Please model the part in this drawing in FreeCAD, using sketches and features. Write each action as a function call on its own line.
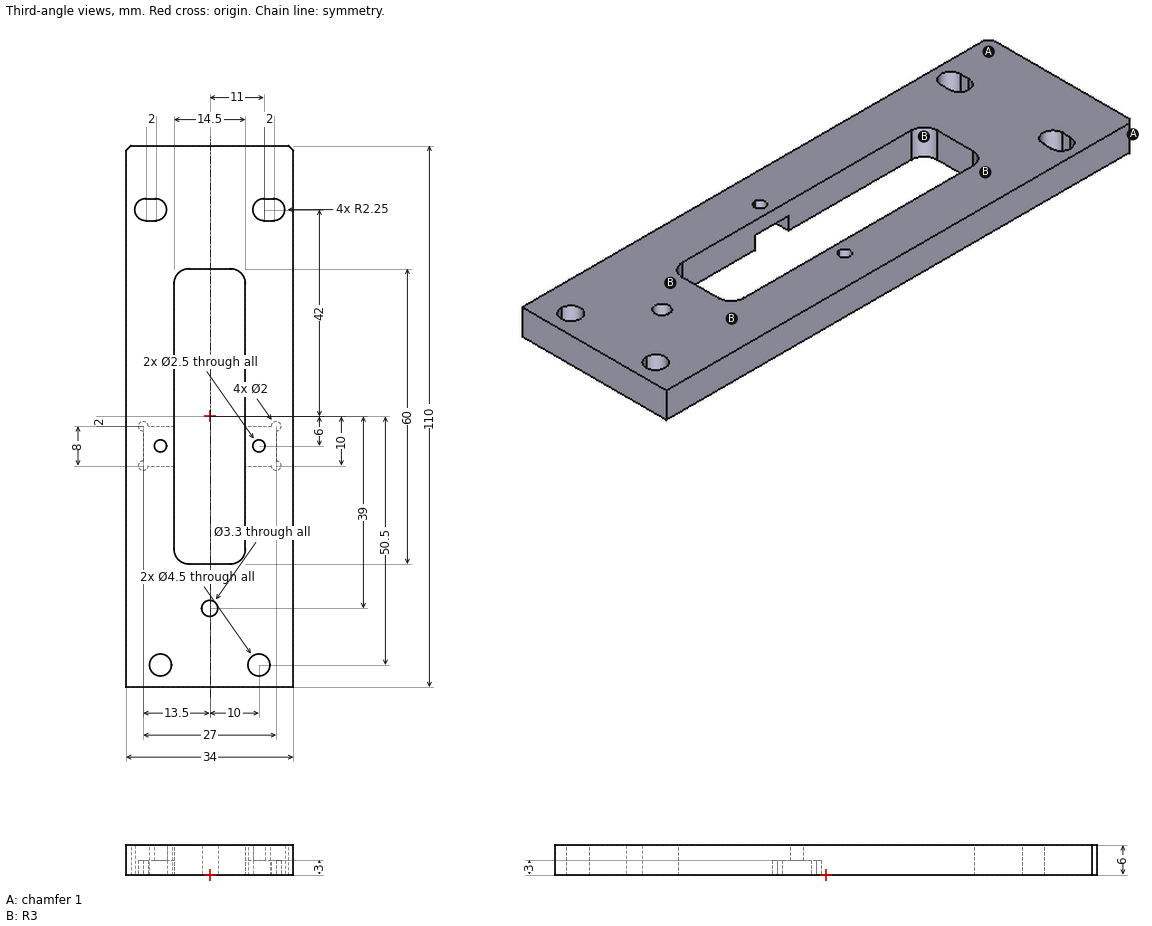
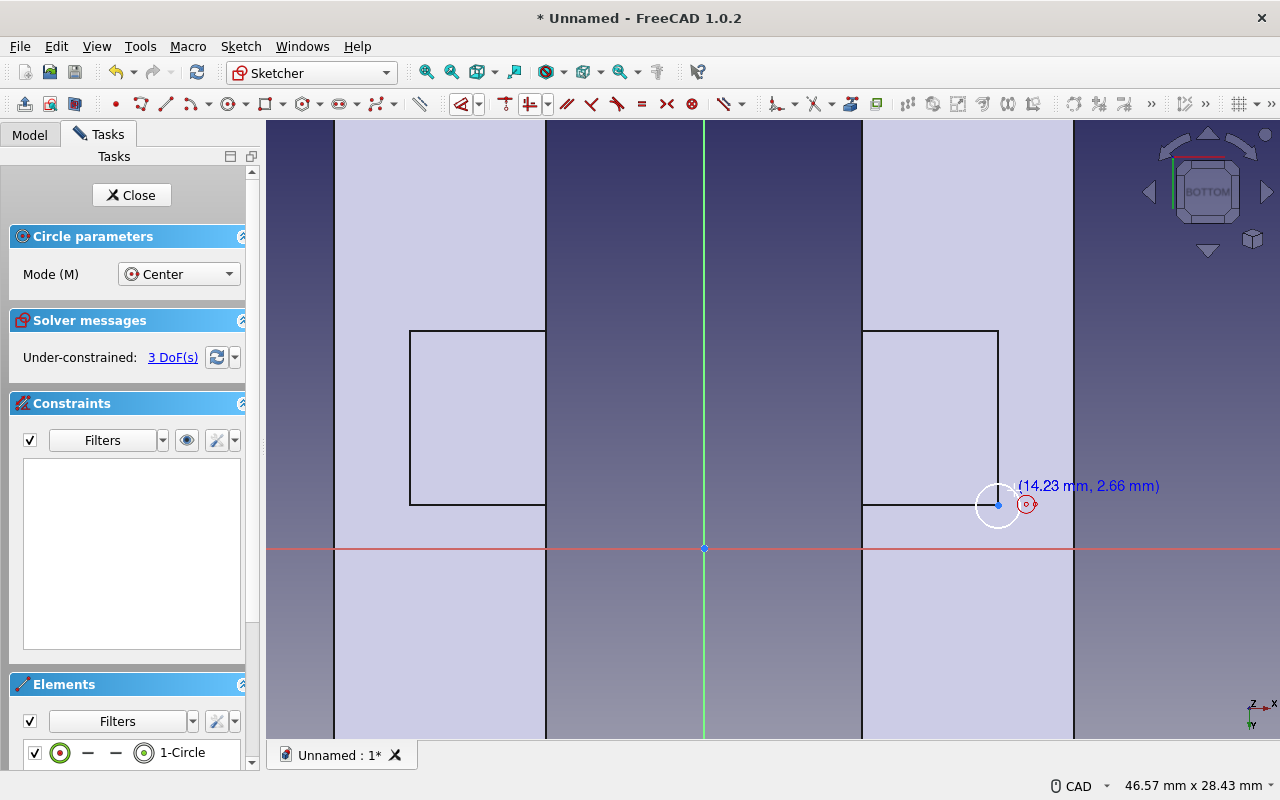
click(998, 331)
click(1014, 316)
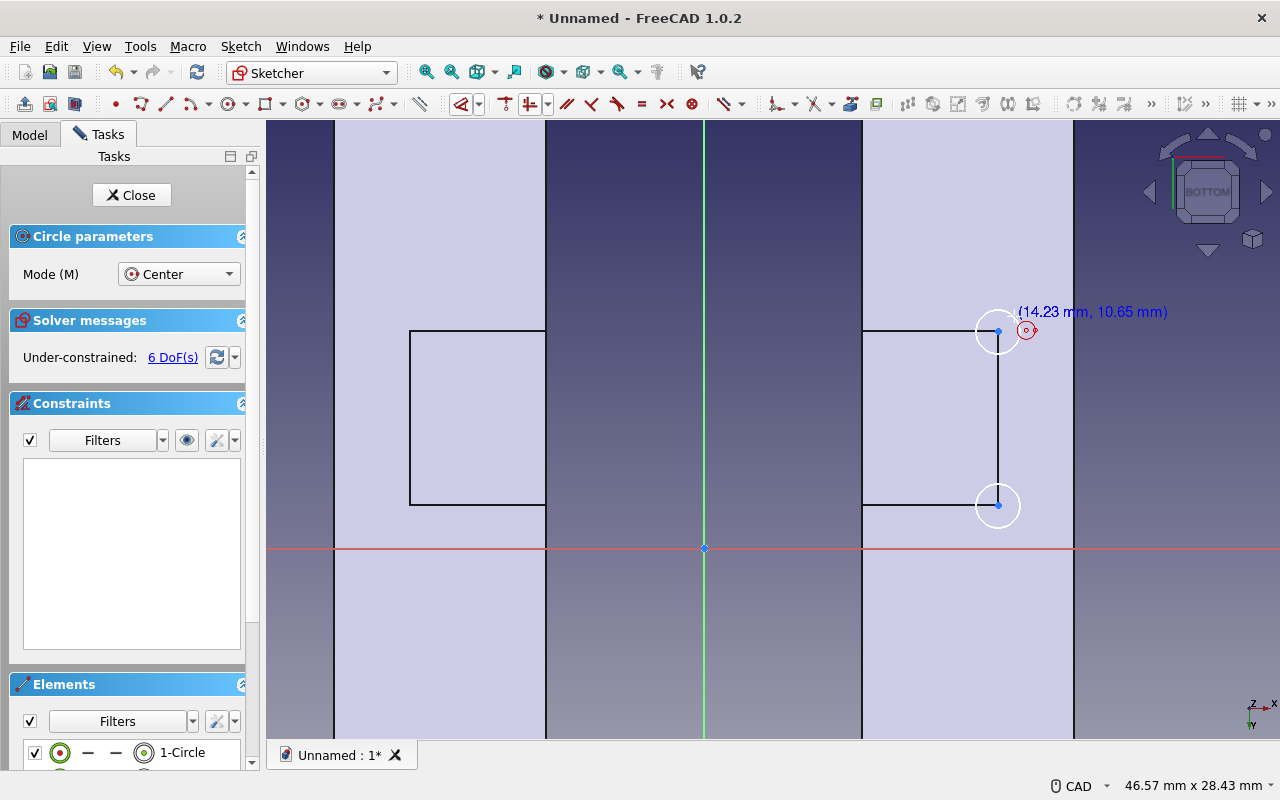
click(410, 331)
click(426, 316)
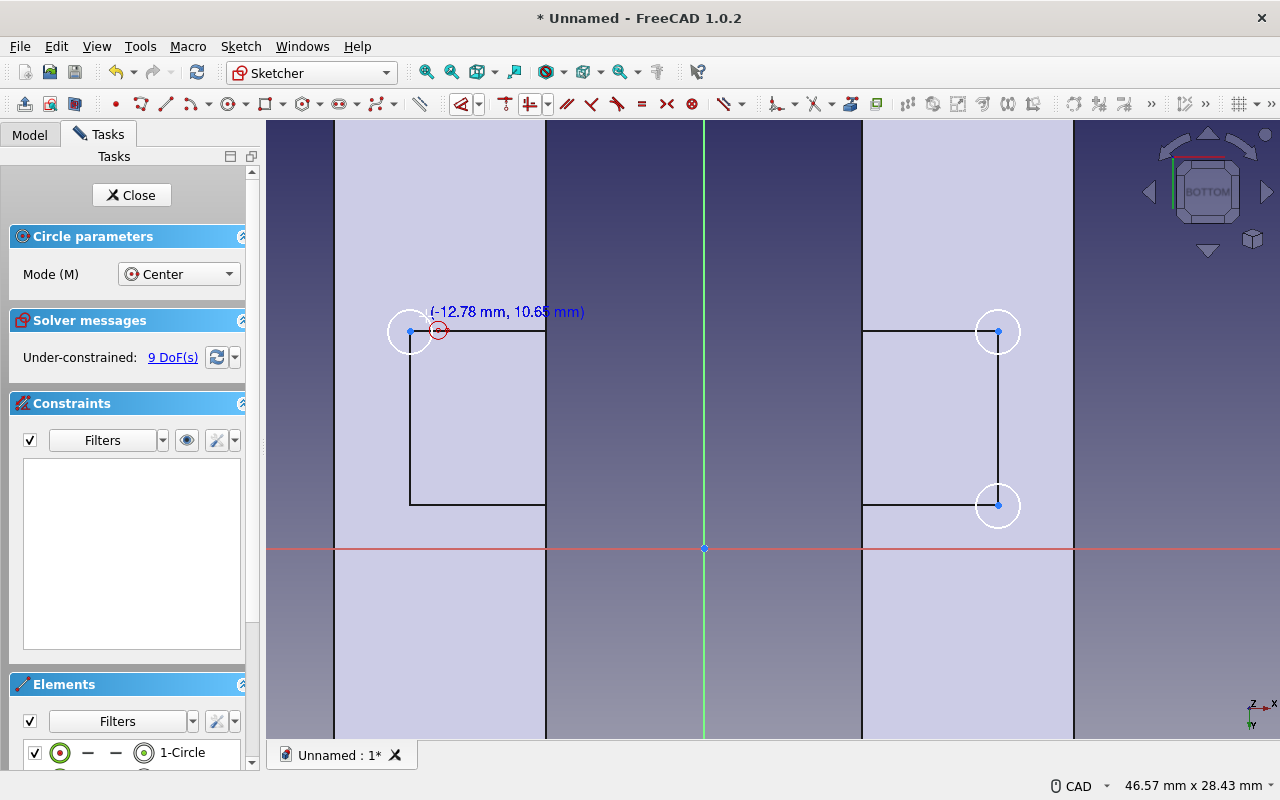
click(410, 505)
click(426, 490)
key(Escape)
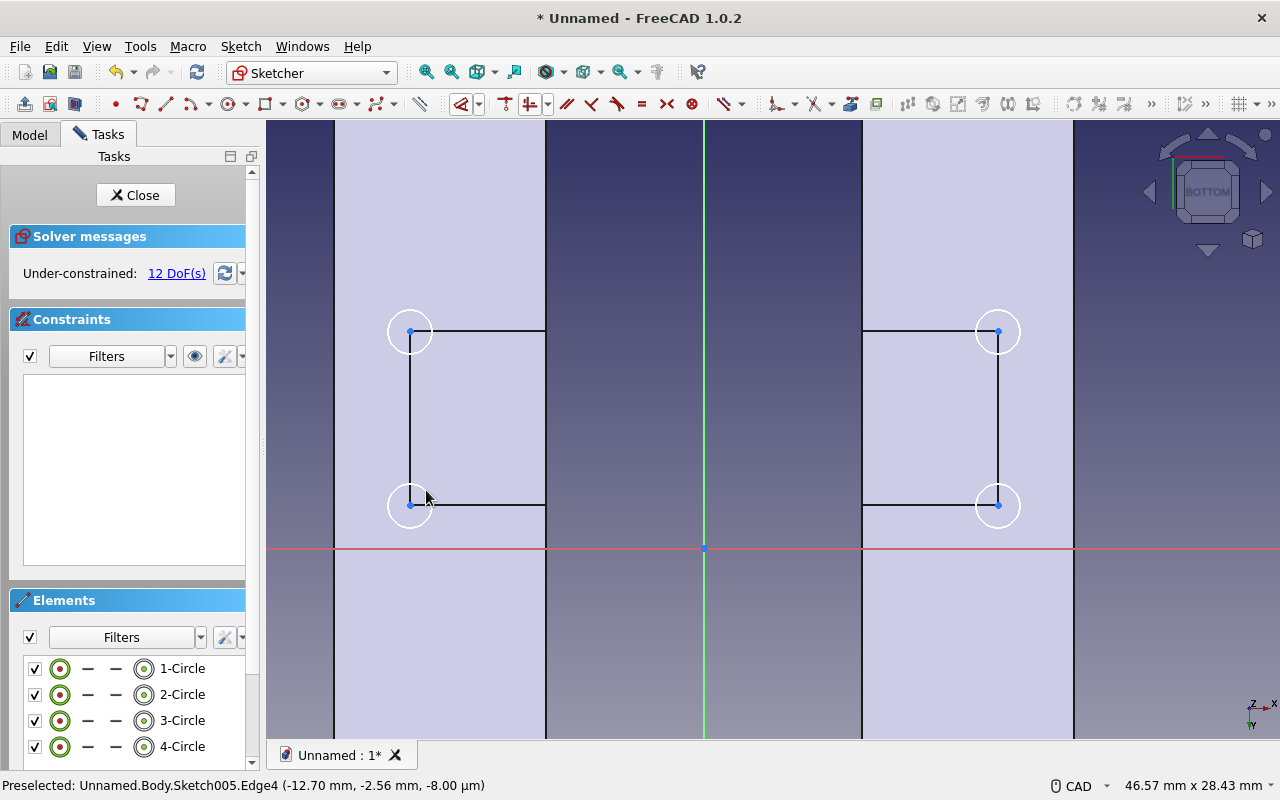
click(1013, 490)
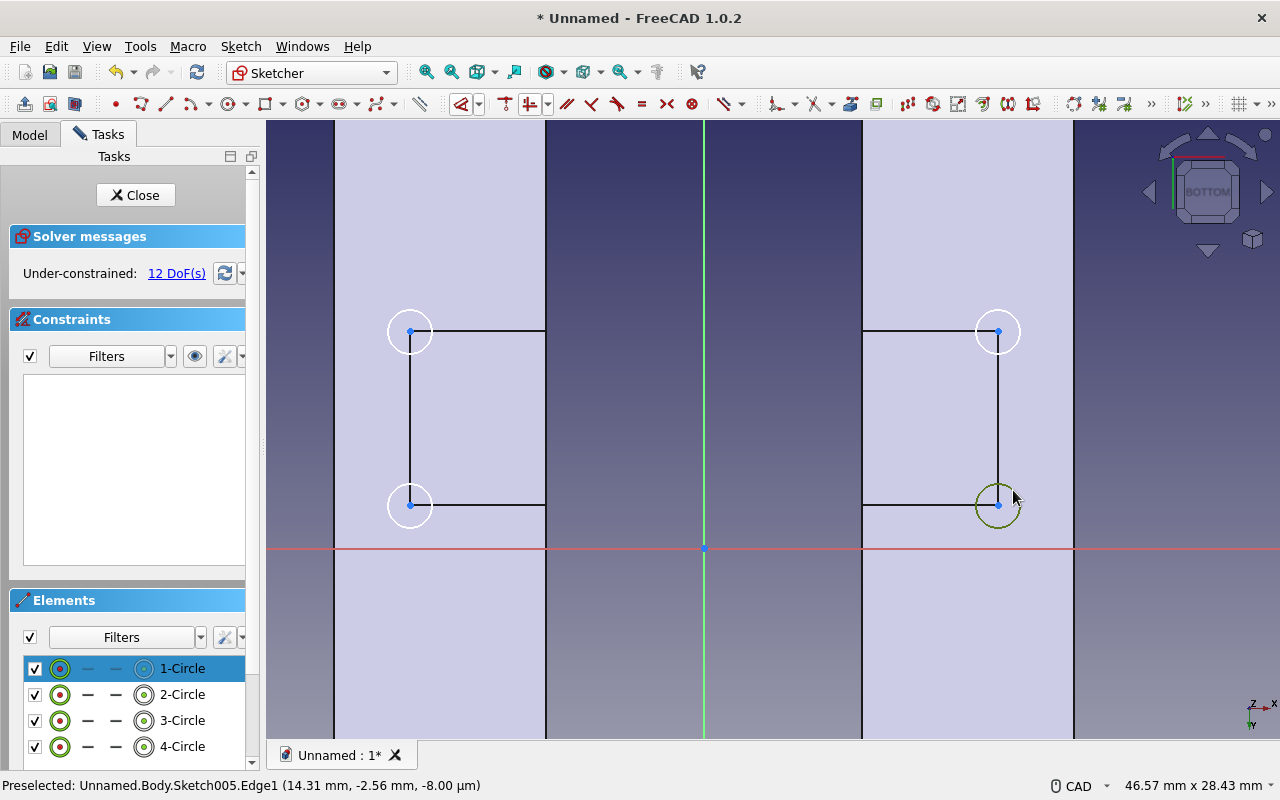
click(1013, 316)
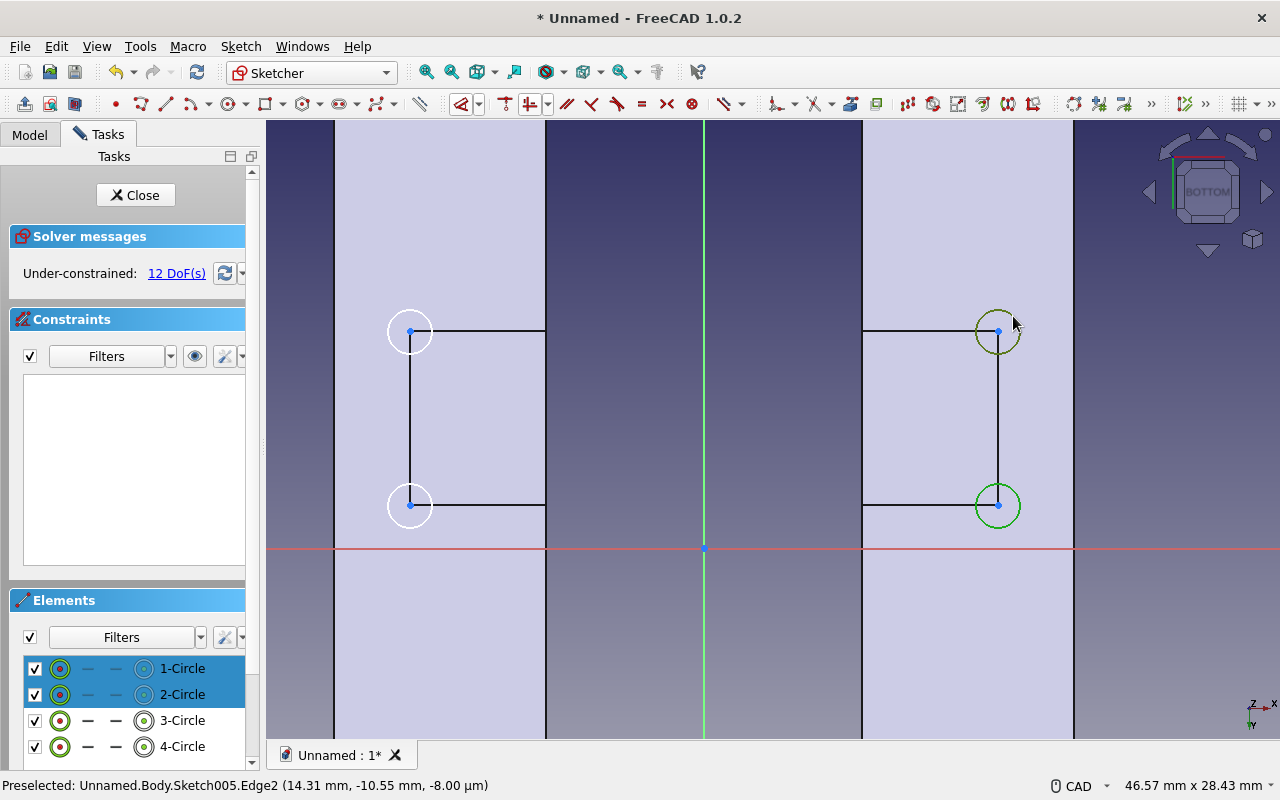
click(425, 316)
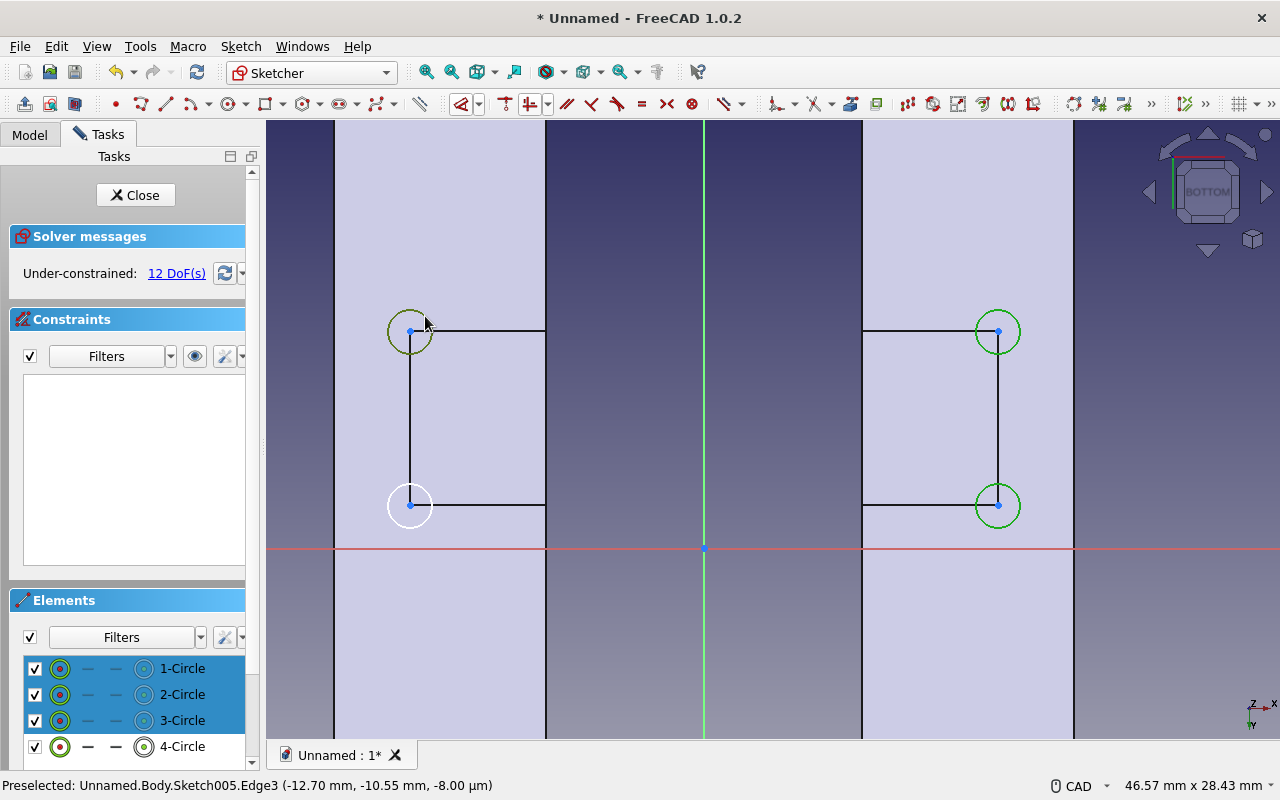
click(425, 490)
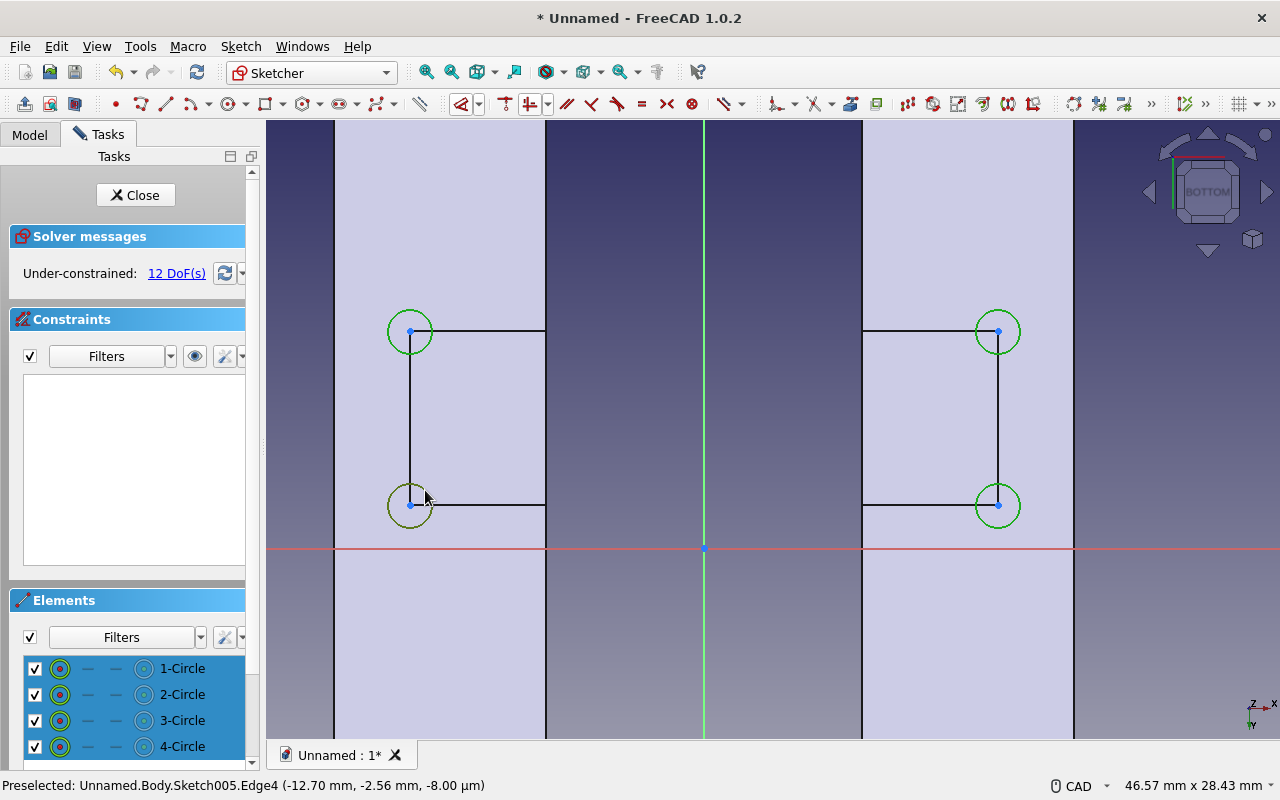
click(642, 104)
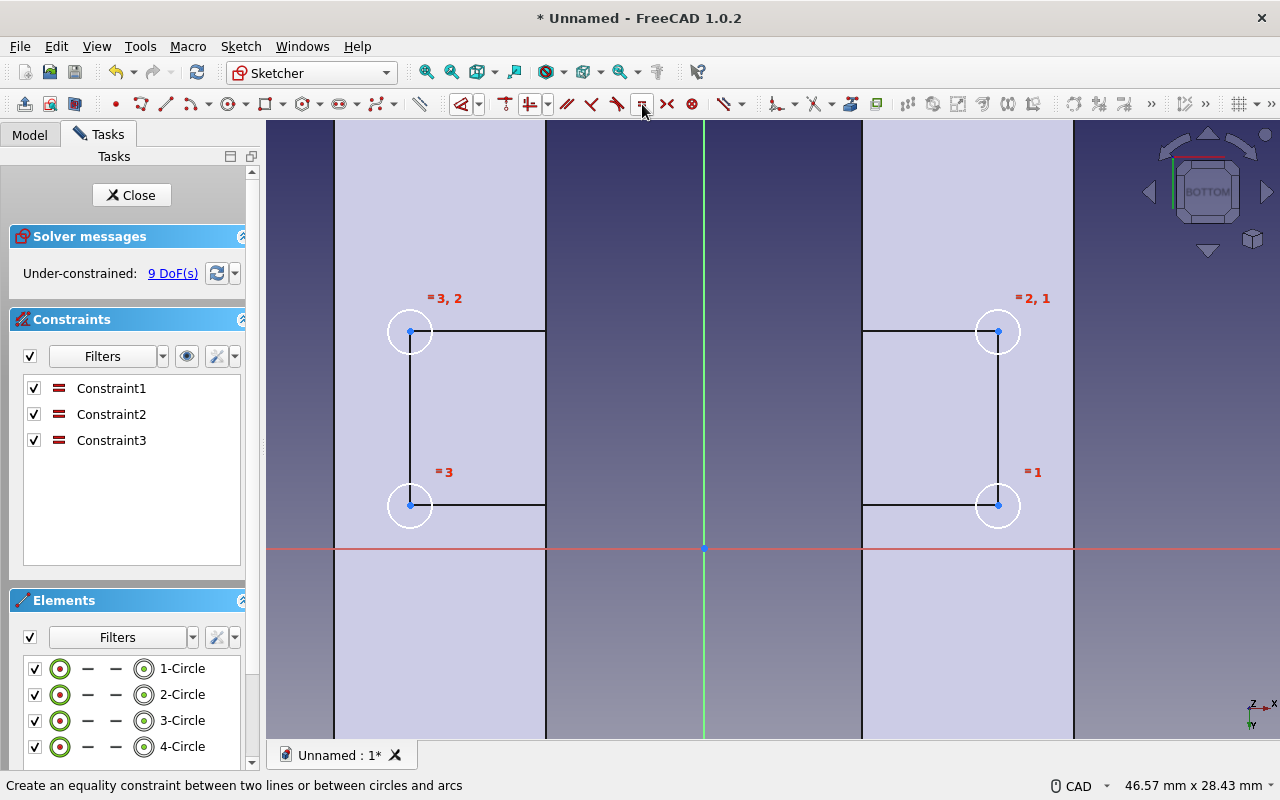
click(998, 332)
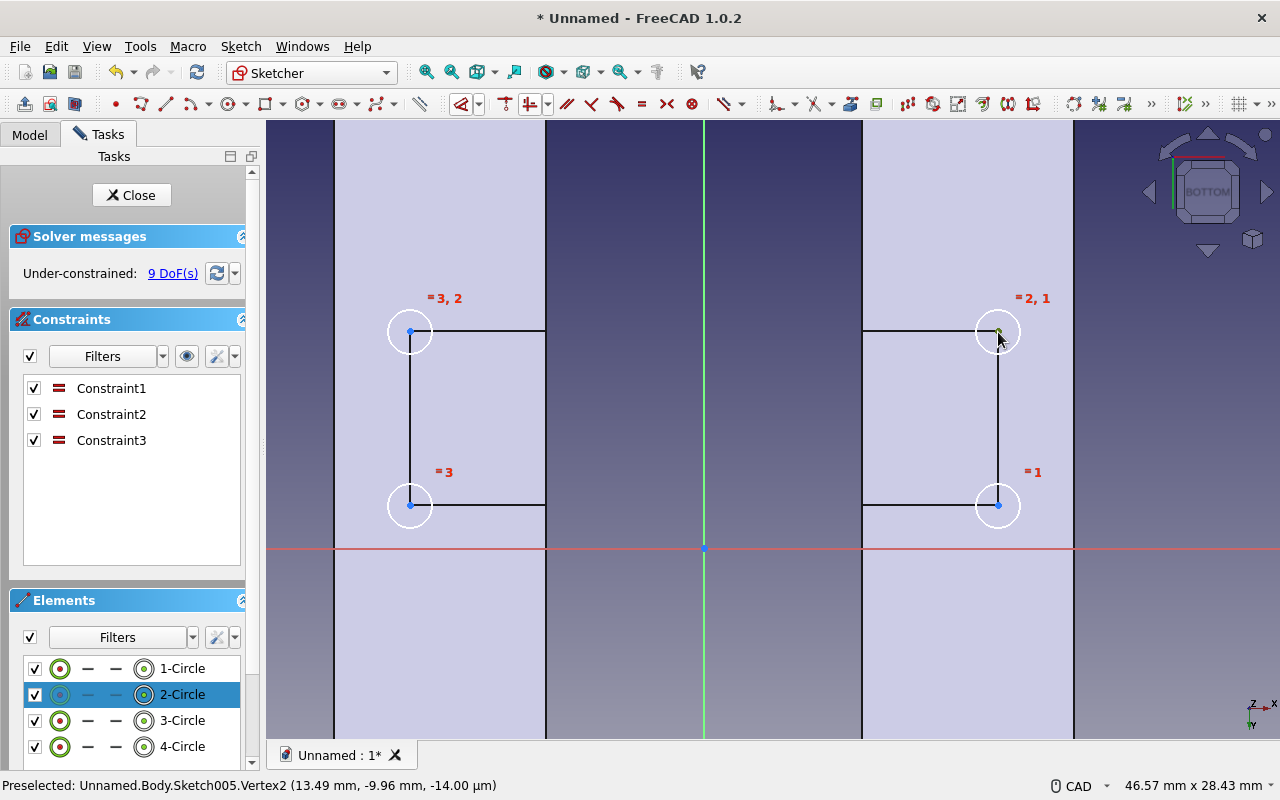
click(410, 332)